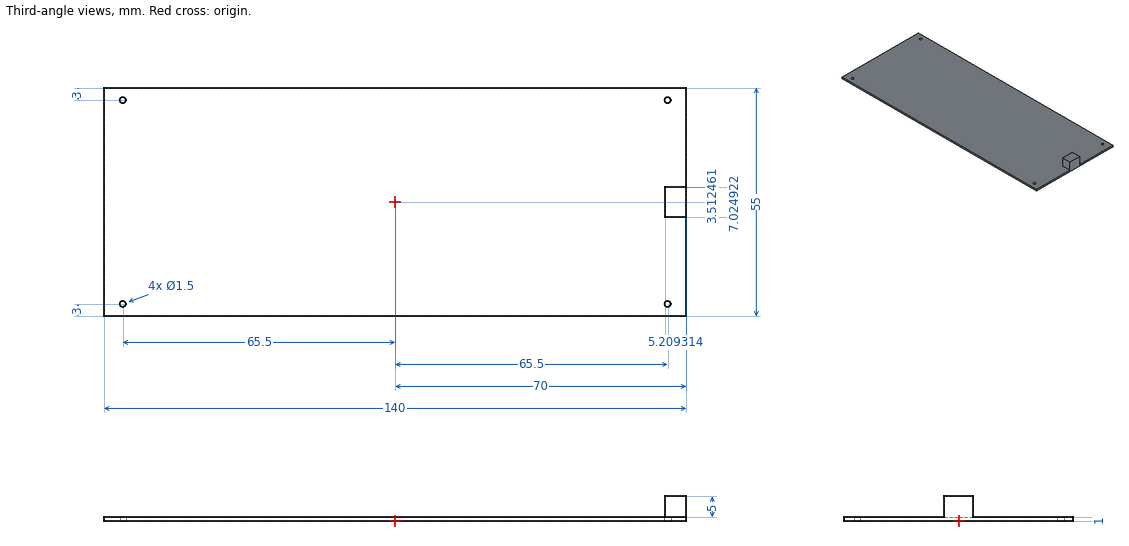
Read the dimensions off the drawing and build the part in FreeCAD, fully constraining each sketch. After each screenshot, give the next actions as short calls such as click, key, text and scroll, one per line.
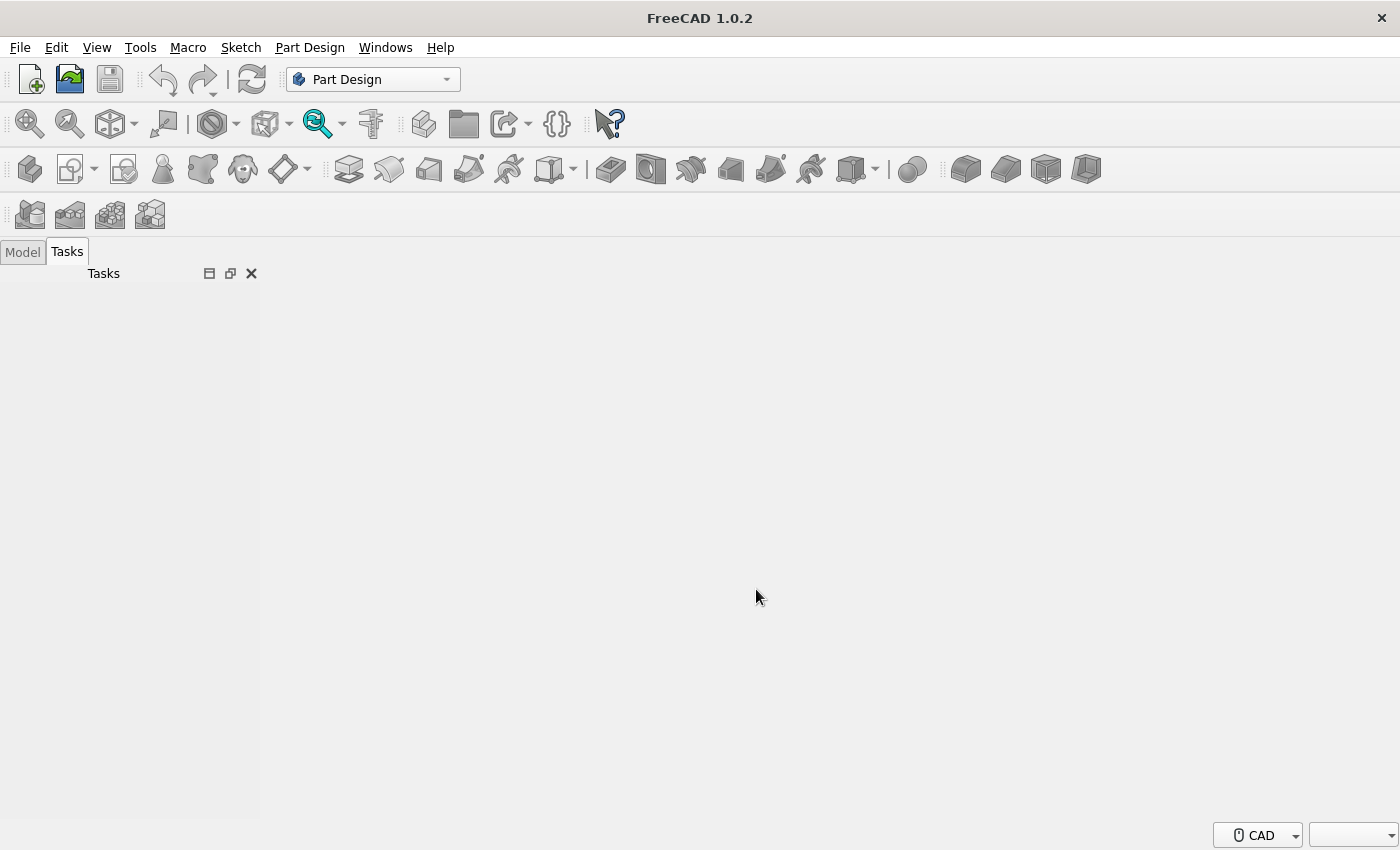
key(ctrl+n)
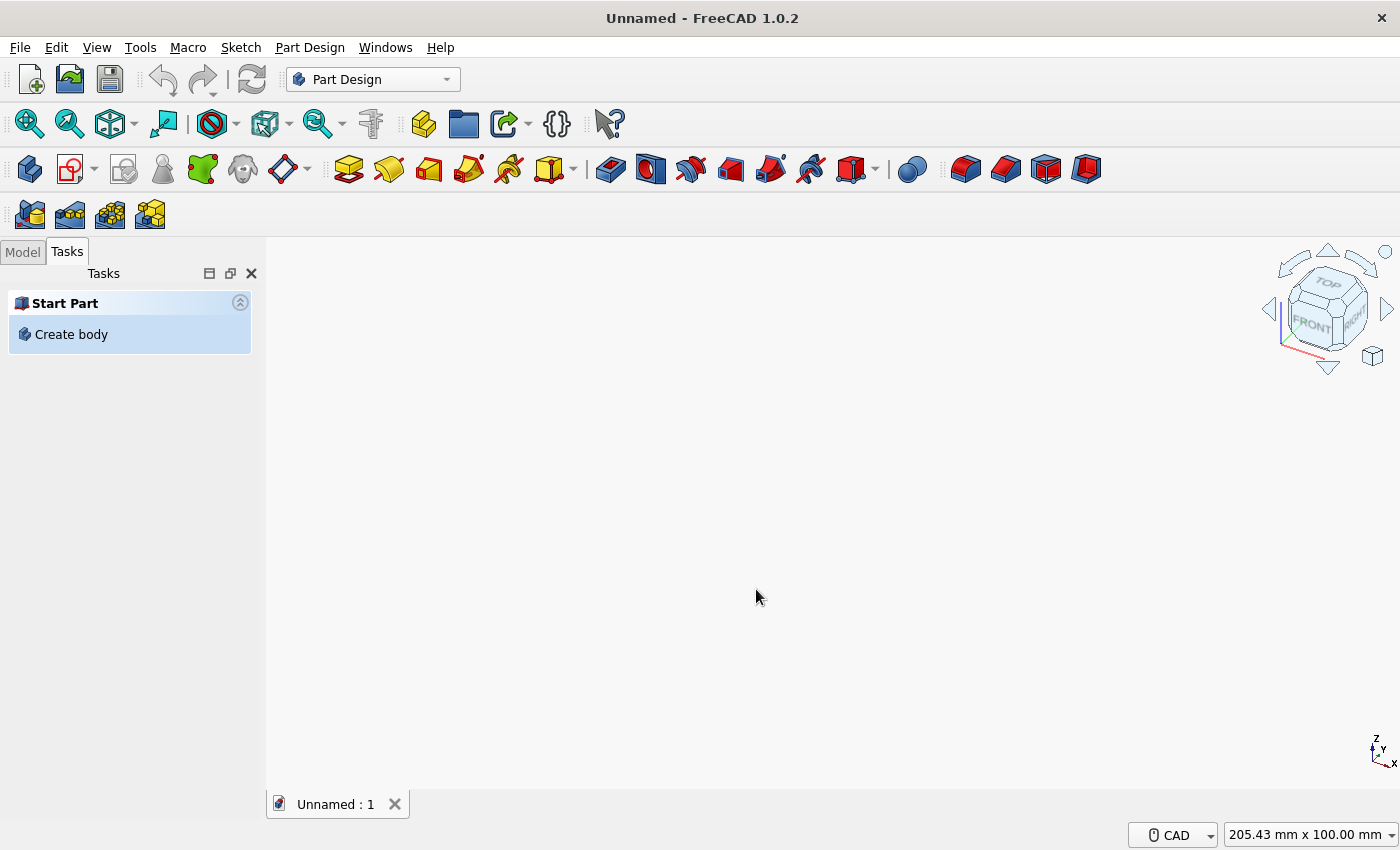
click(70, 170)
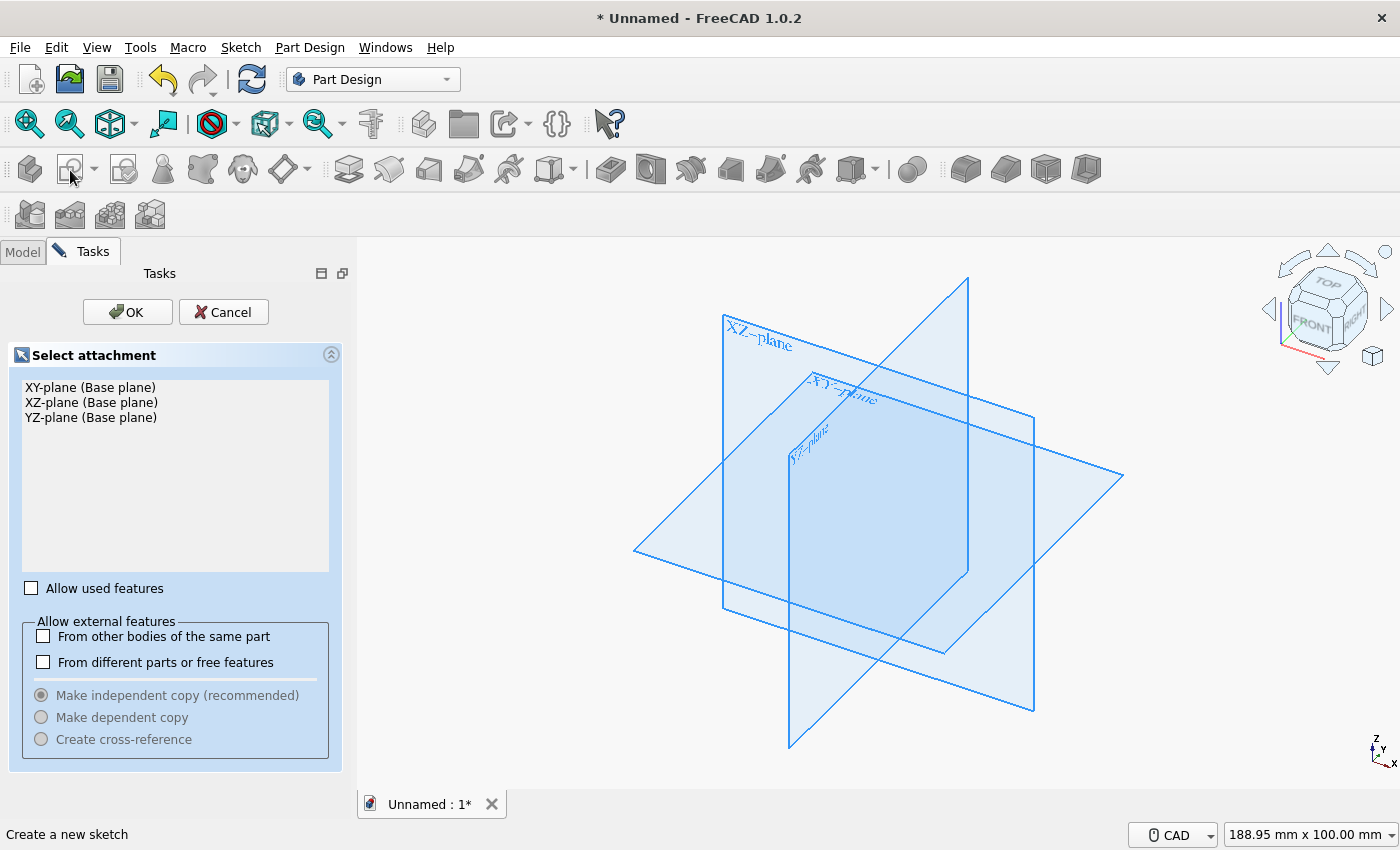
click(82, 388)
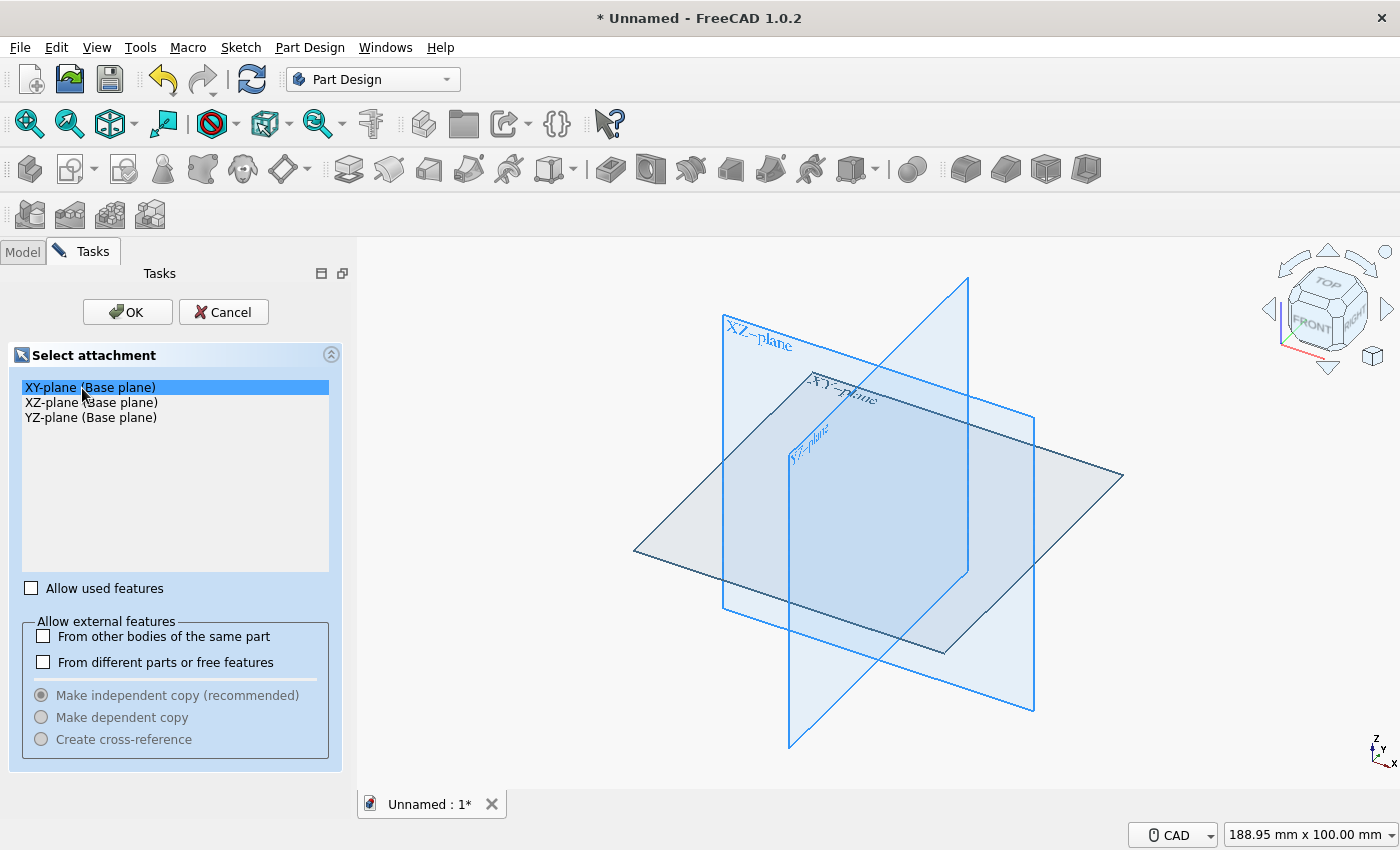
click(128, 312)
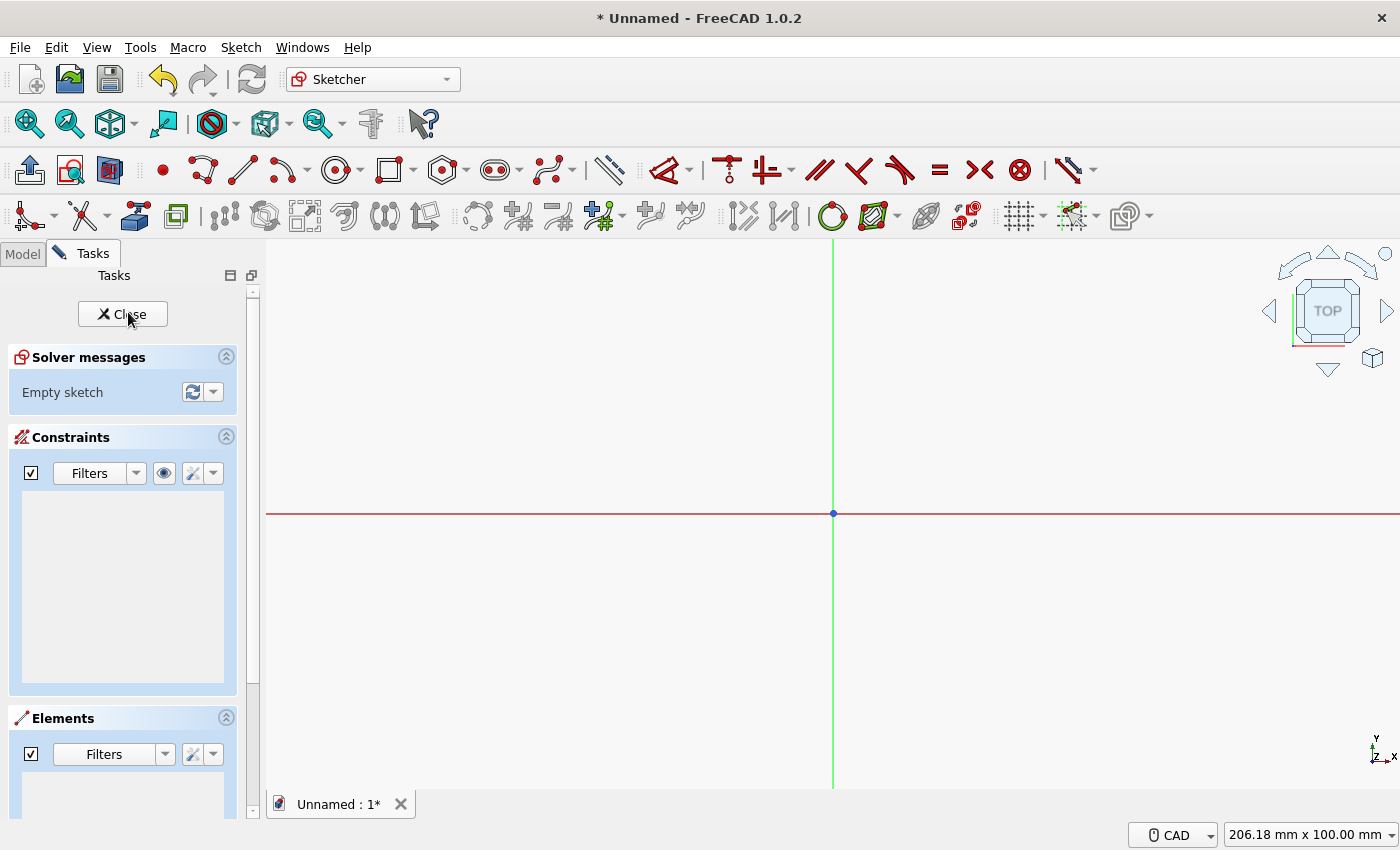
scroll(455, 514, down, 1)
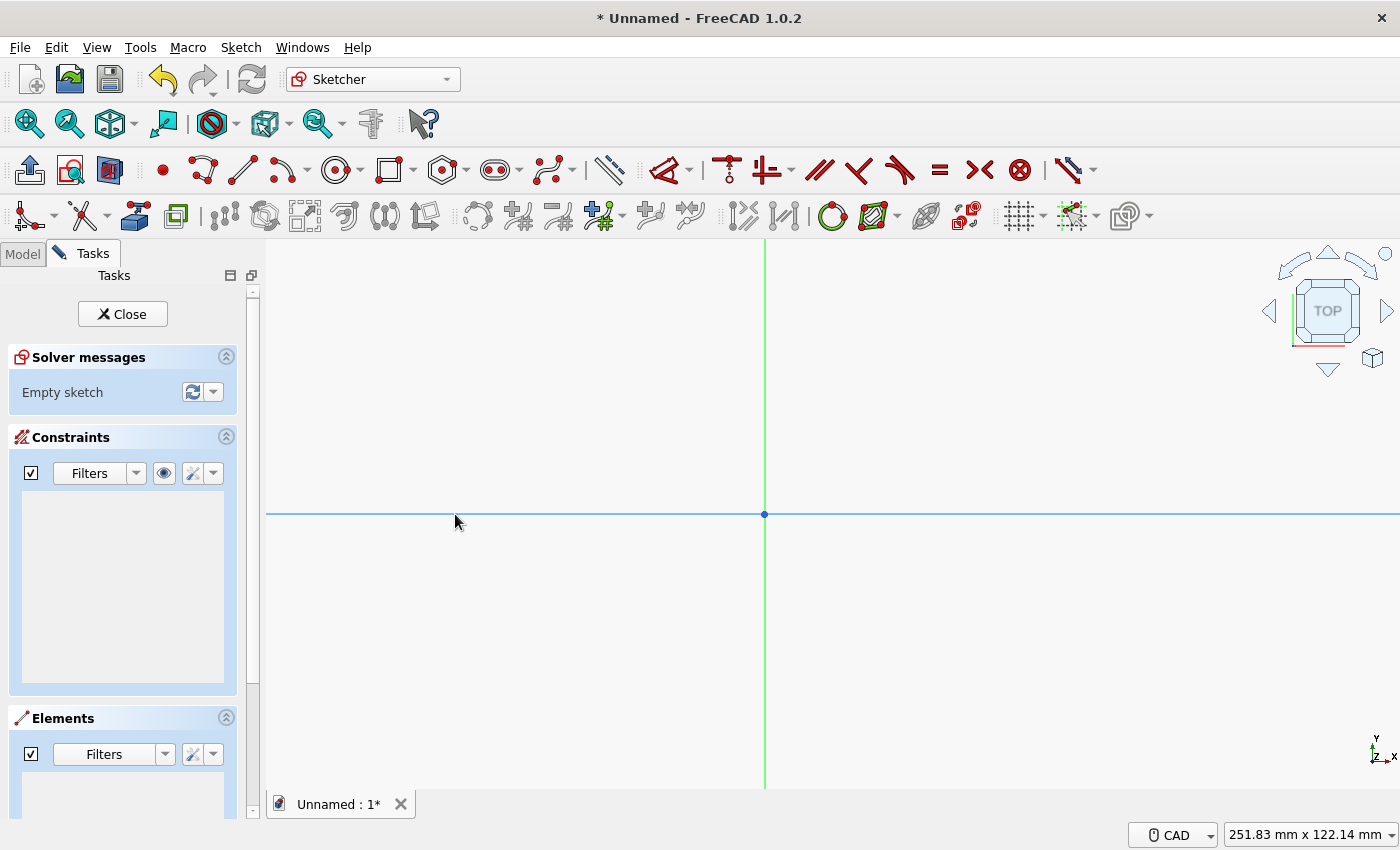
key(g)
key(v)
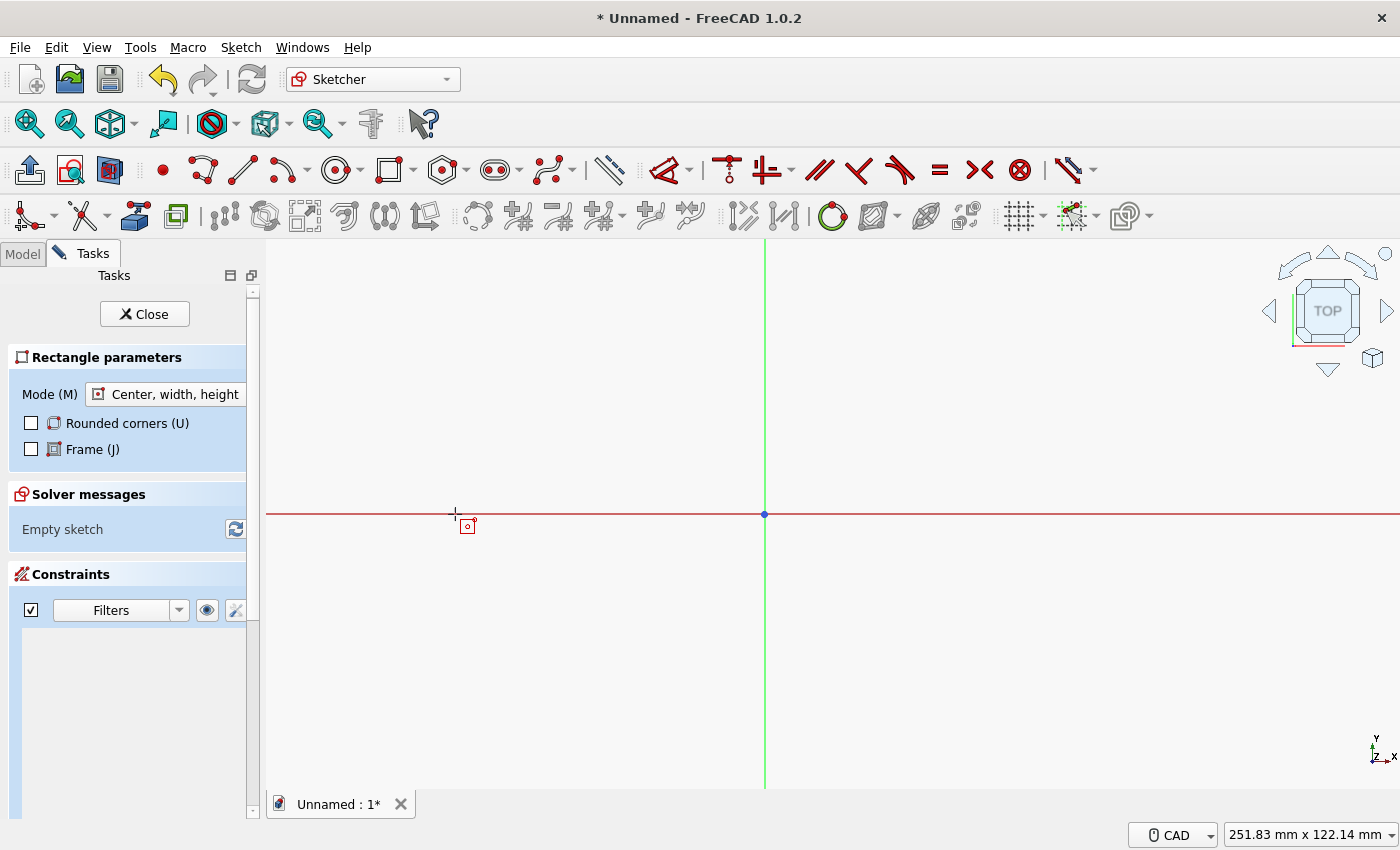
click(765, 514)
move(1080, 390)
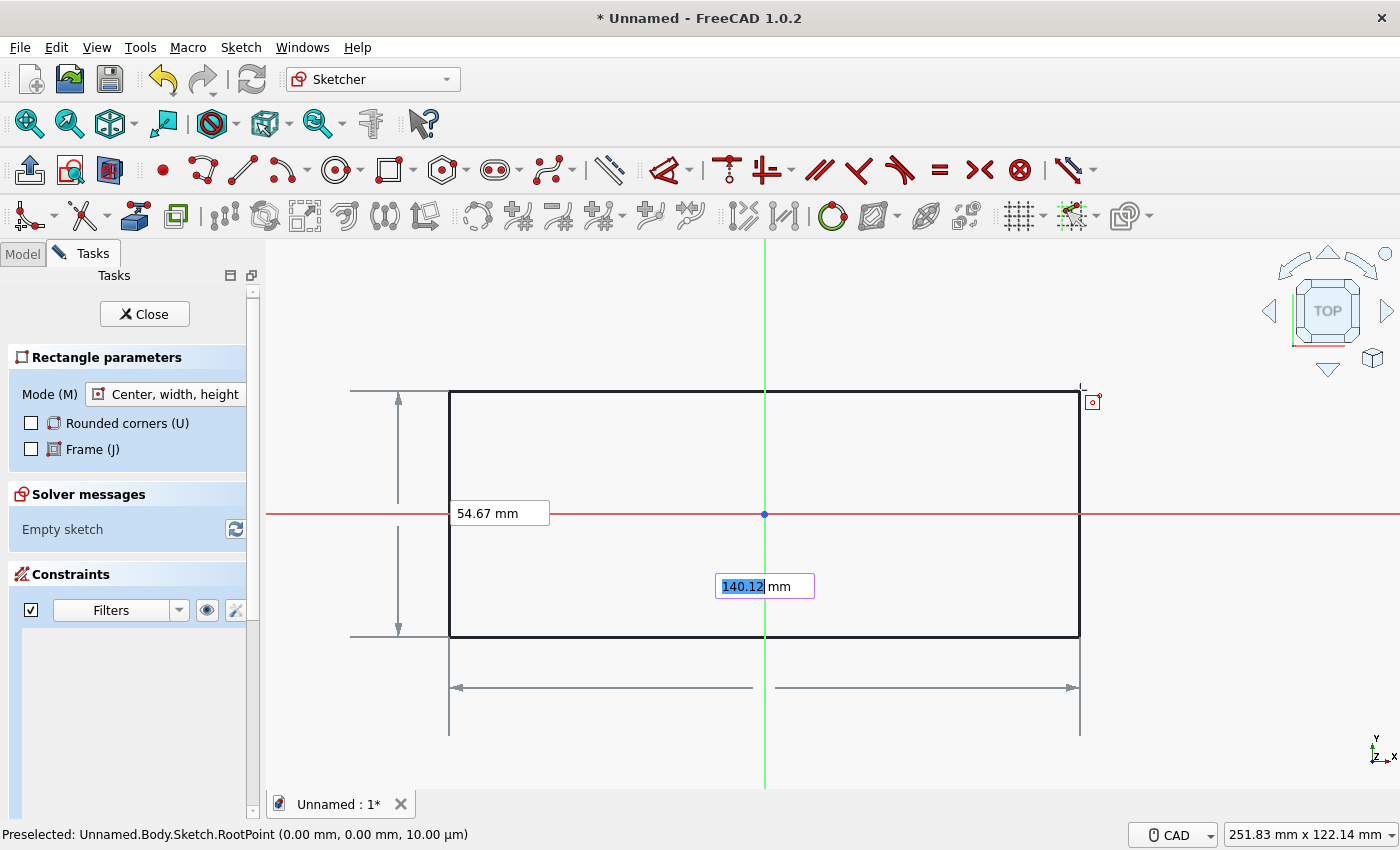
text(140)
key(Tab)
text(55)
key(Return)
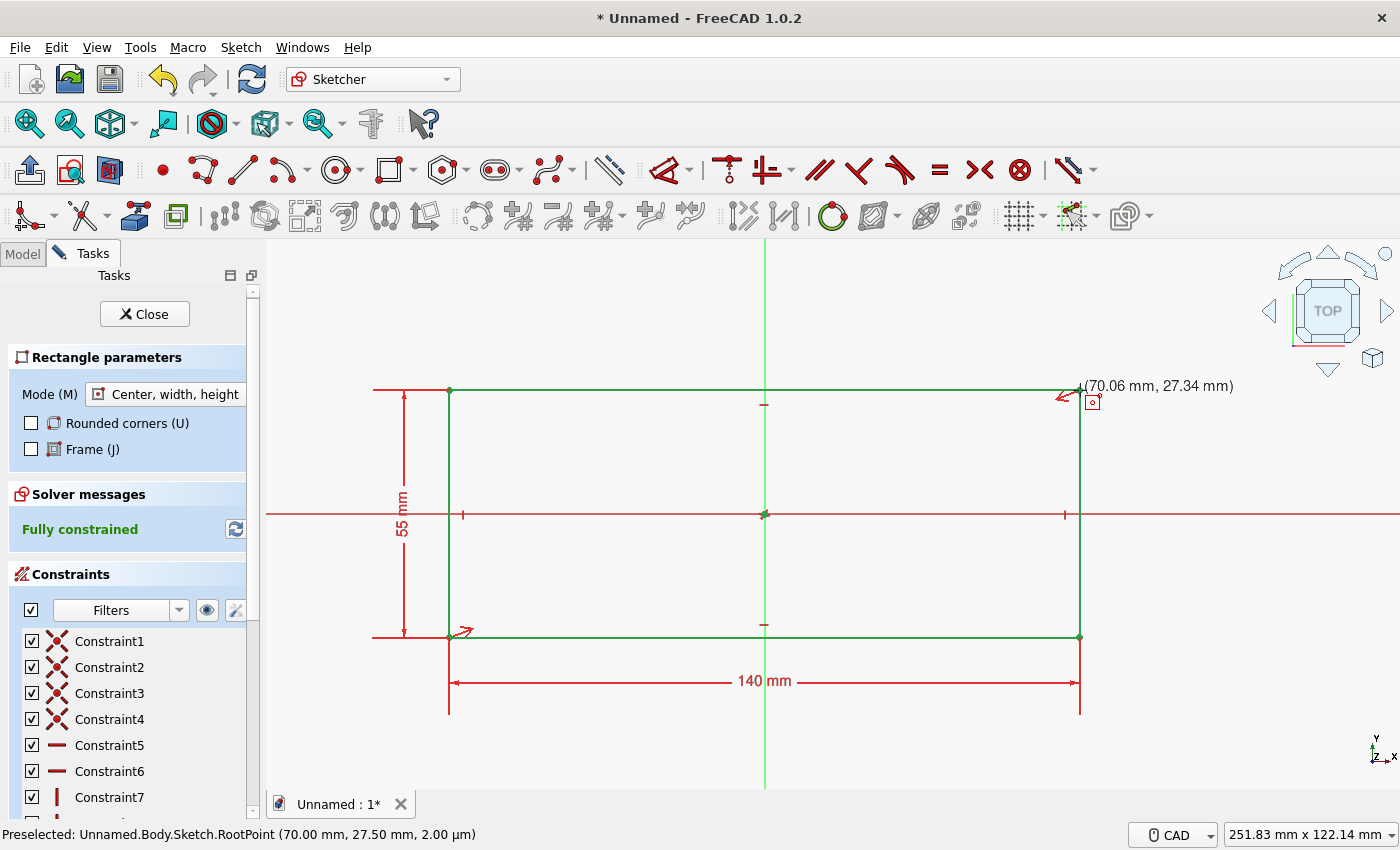
click(336, 170)